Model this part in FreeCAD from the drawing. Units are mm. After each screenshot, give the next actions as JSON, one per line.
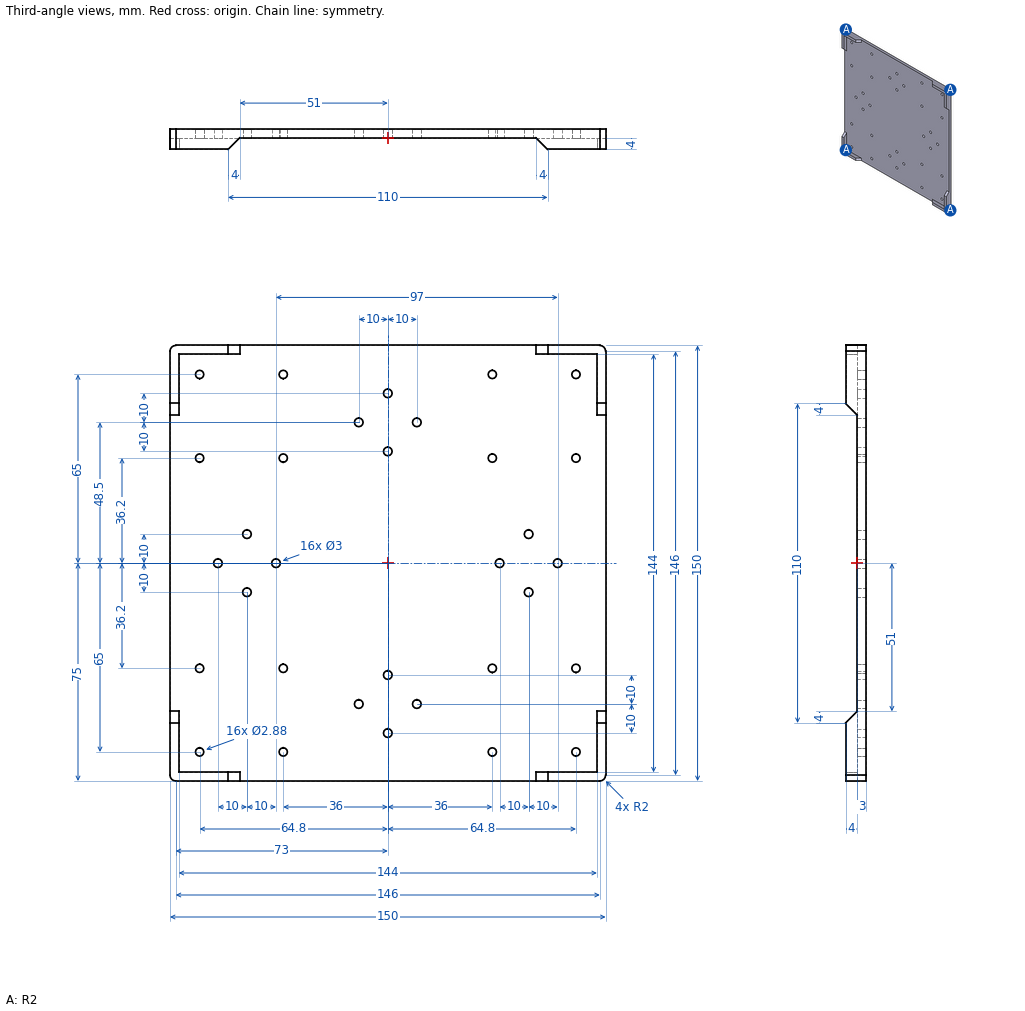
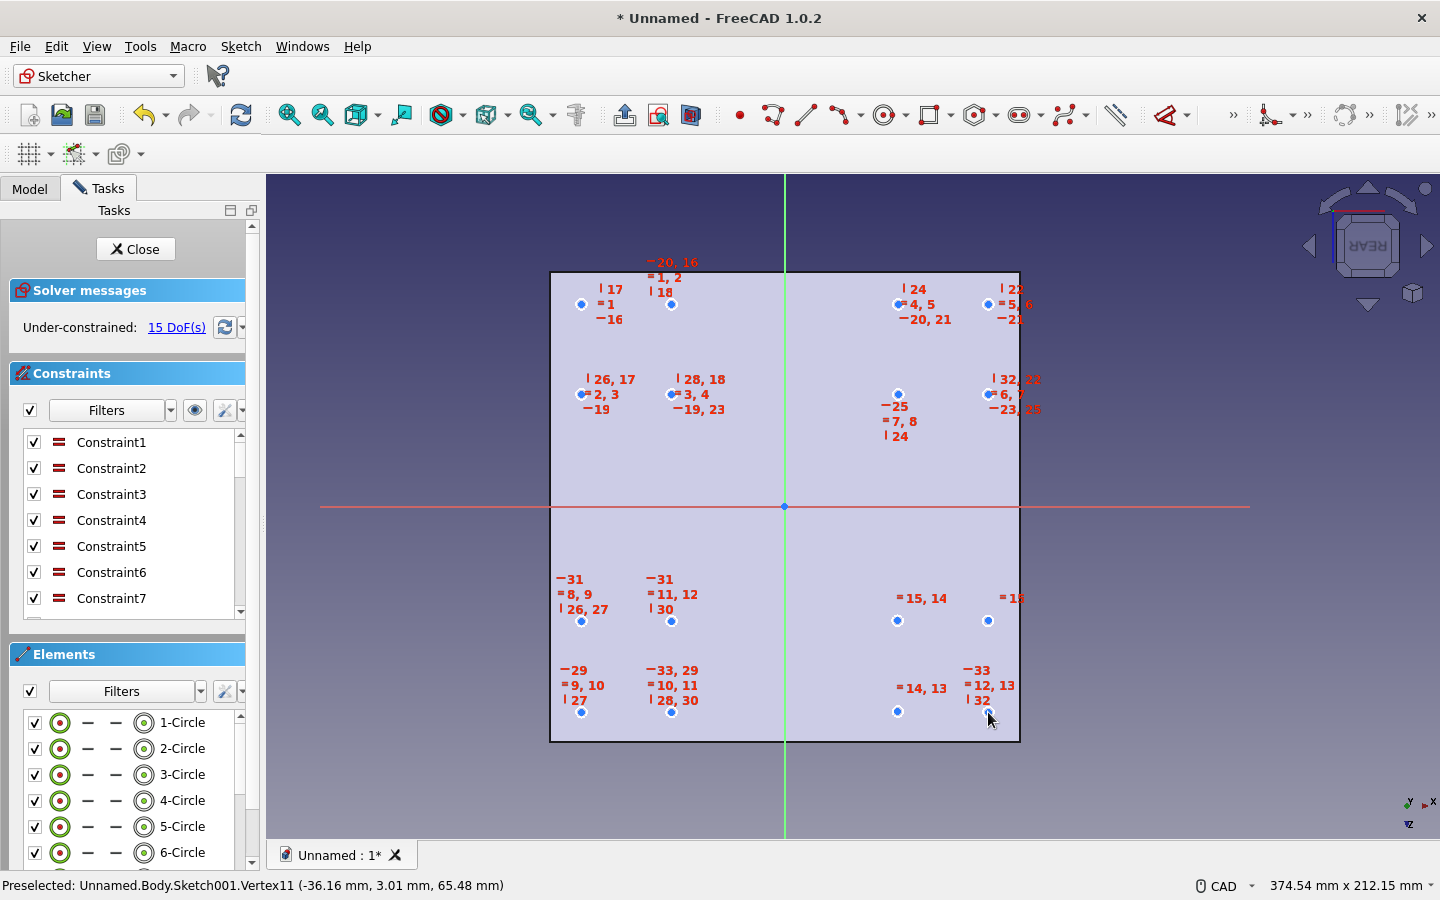
{"action": "left_click", "coordinate": [898, 394]}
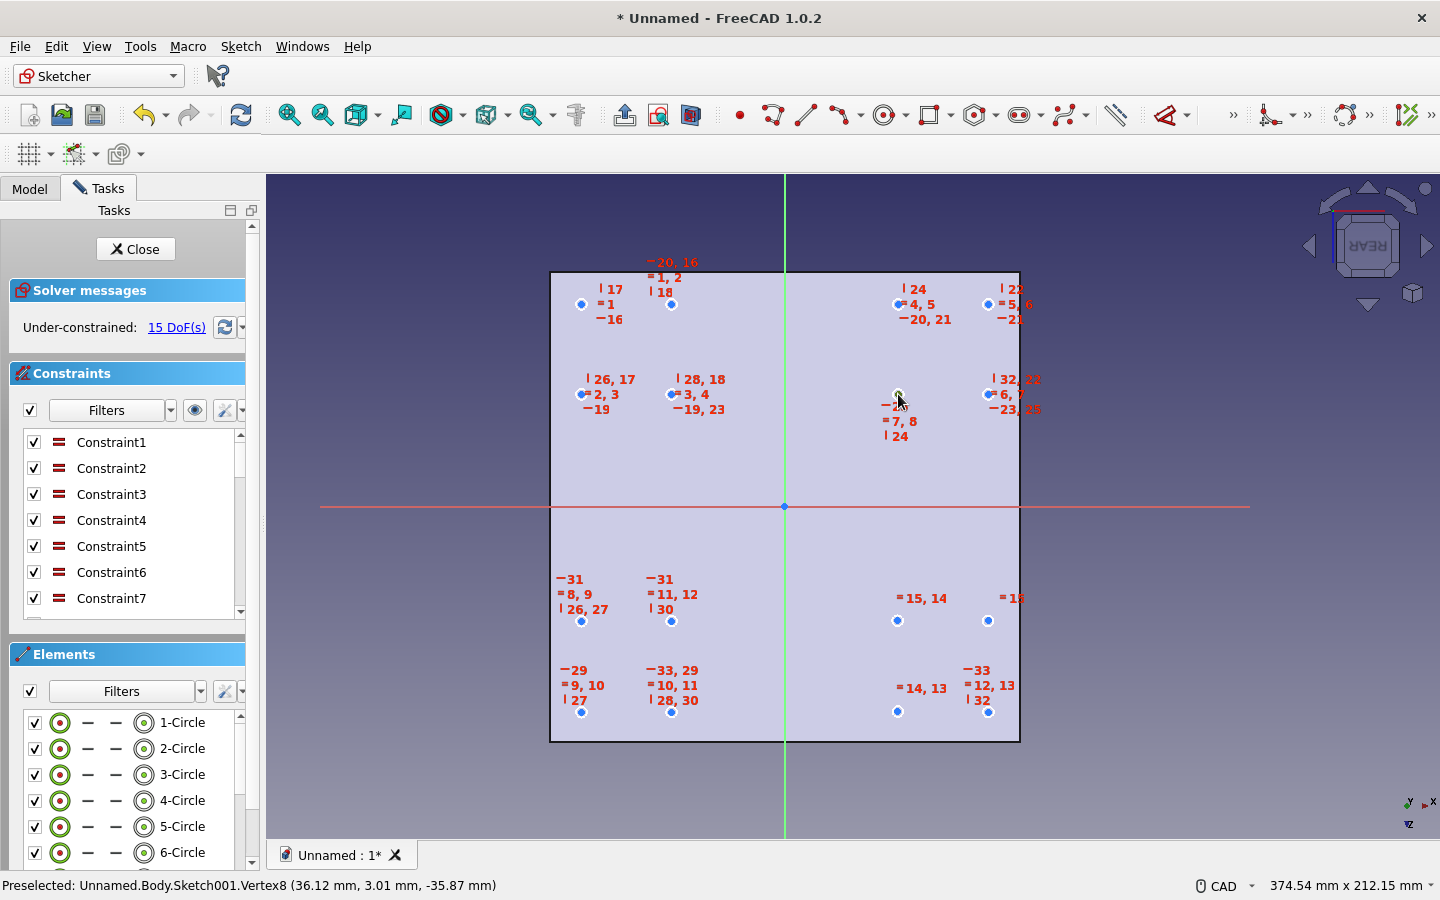
{"action": "left_click", "coordinate": [898, 712]}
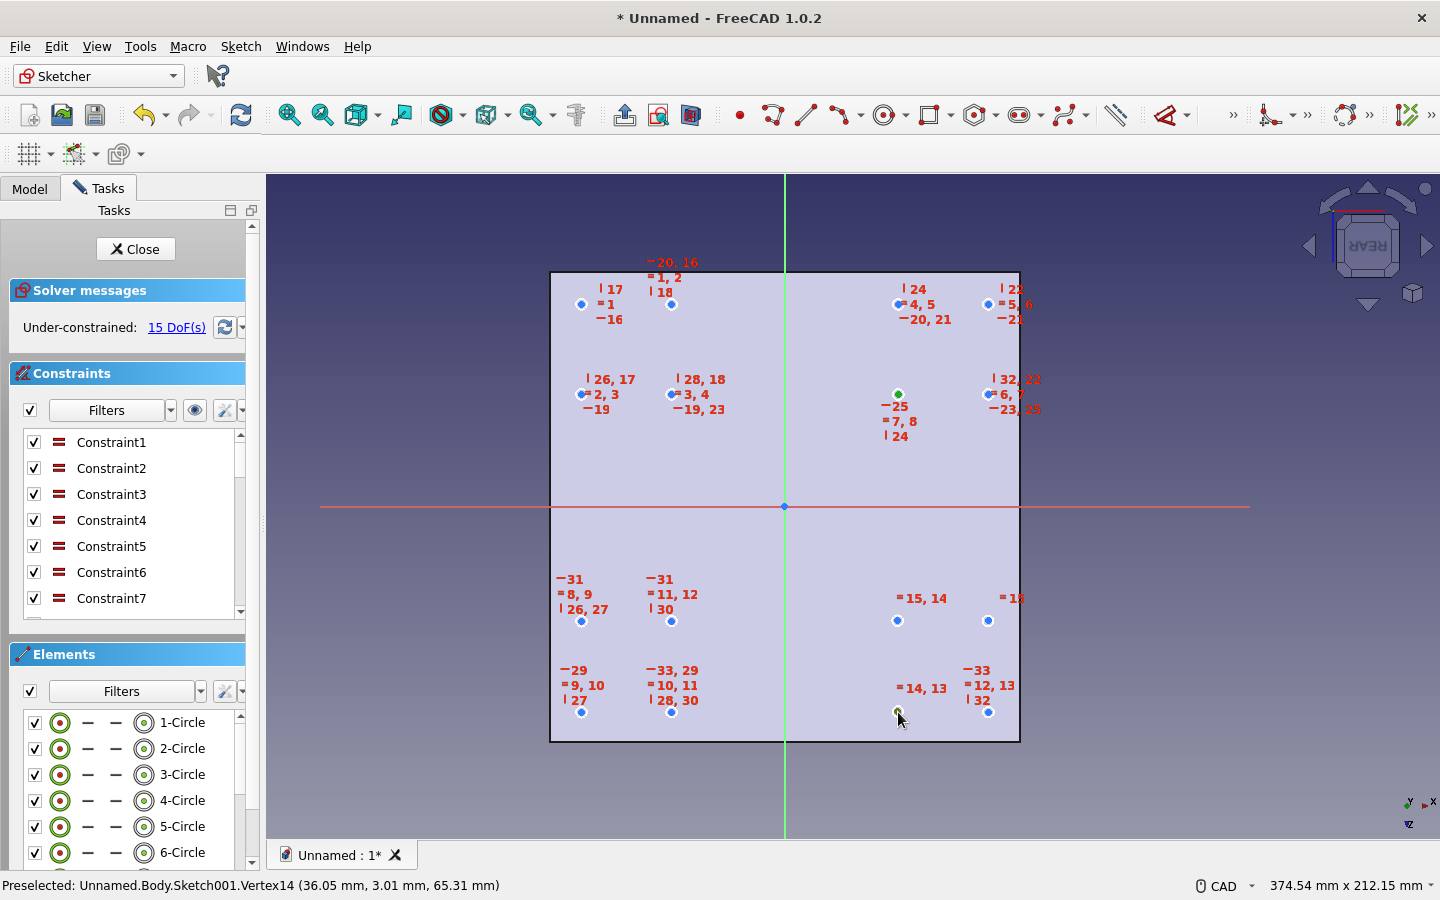
{"action": "key", "text": "v"}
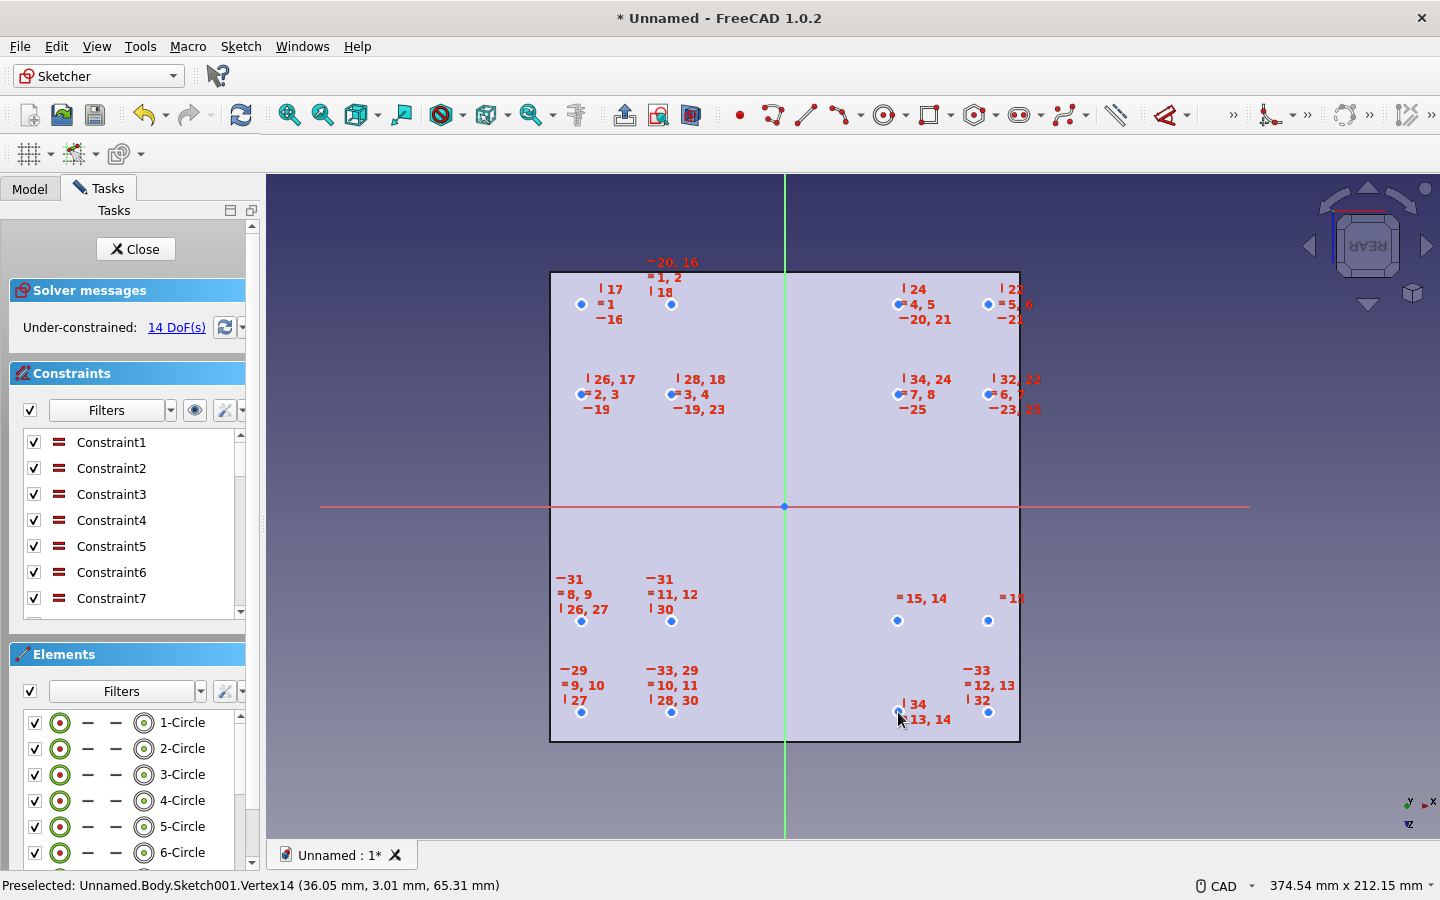
{"action": "left_click", "coordinate": [988, 712]}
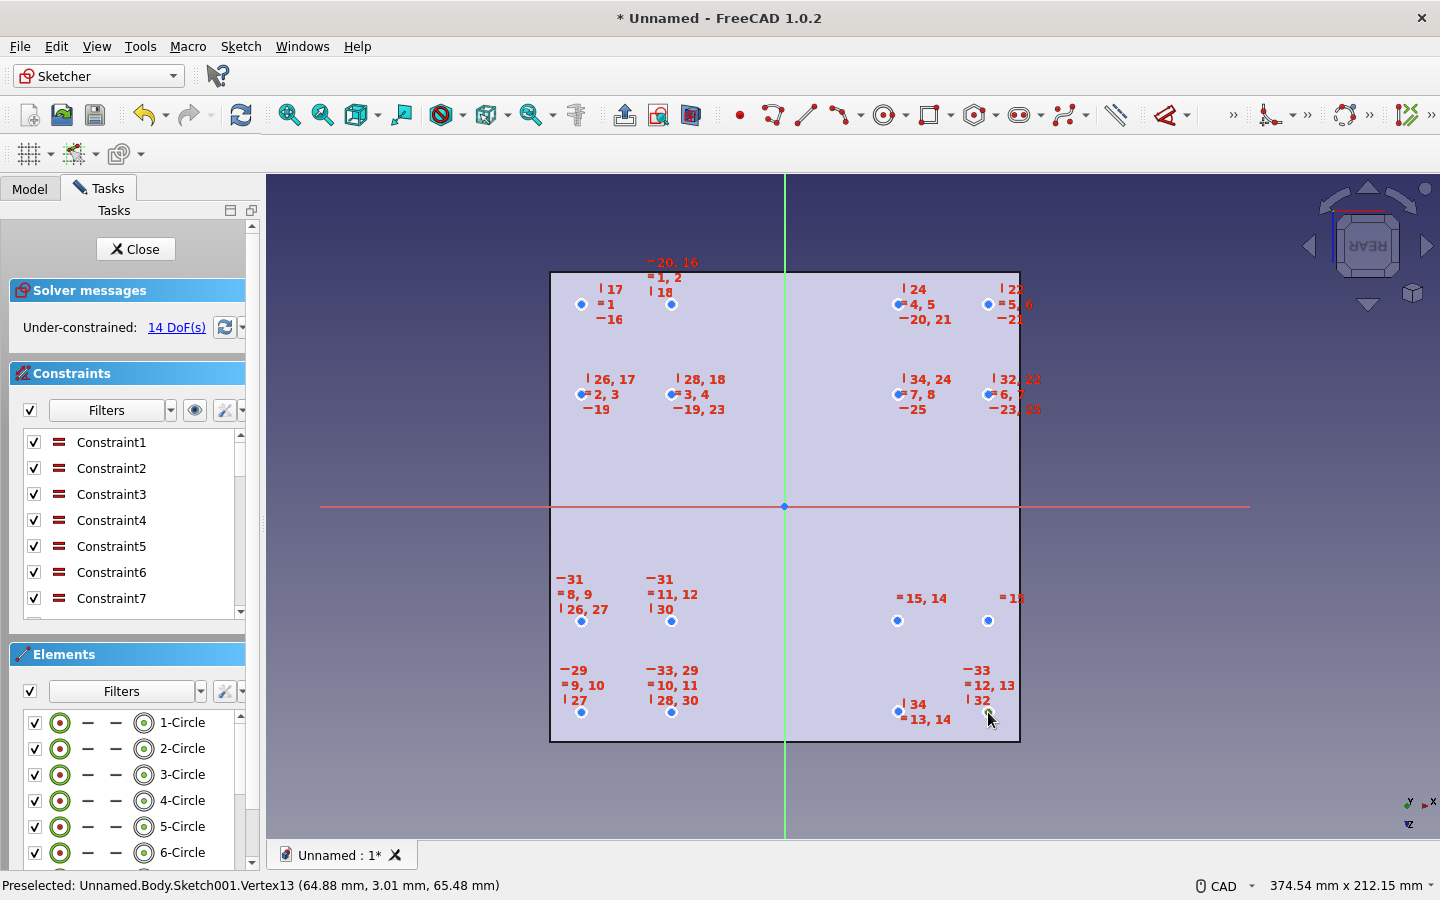
{"action": "left_click", "coordinate": [898, 712]}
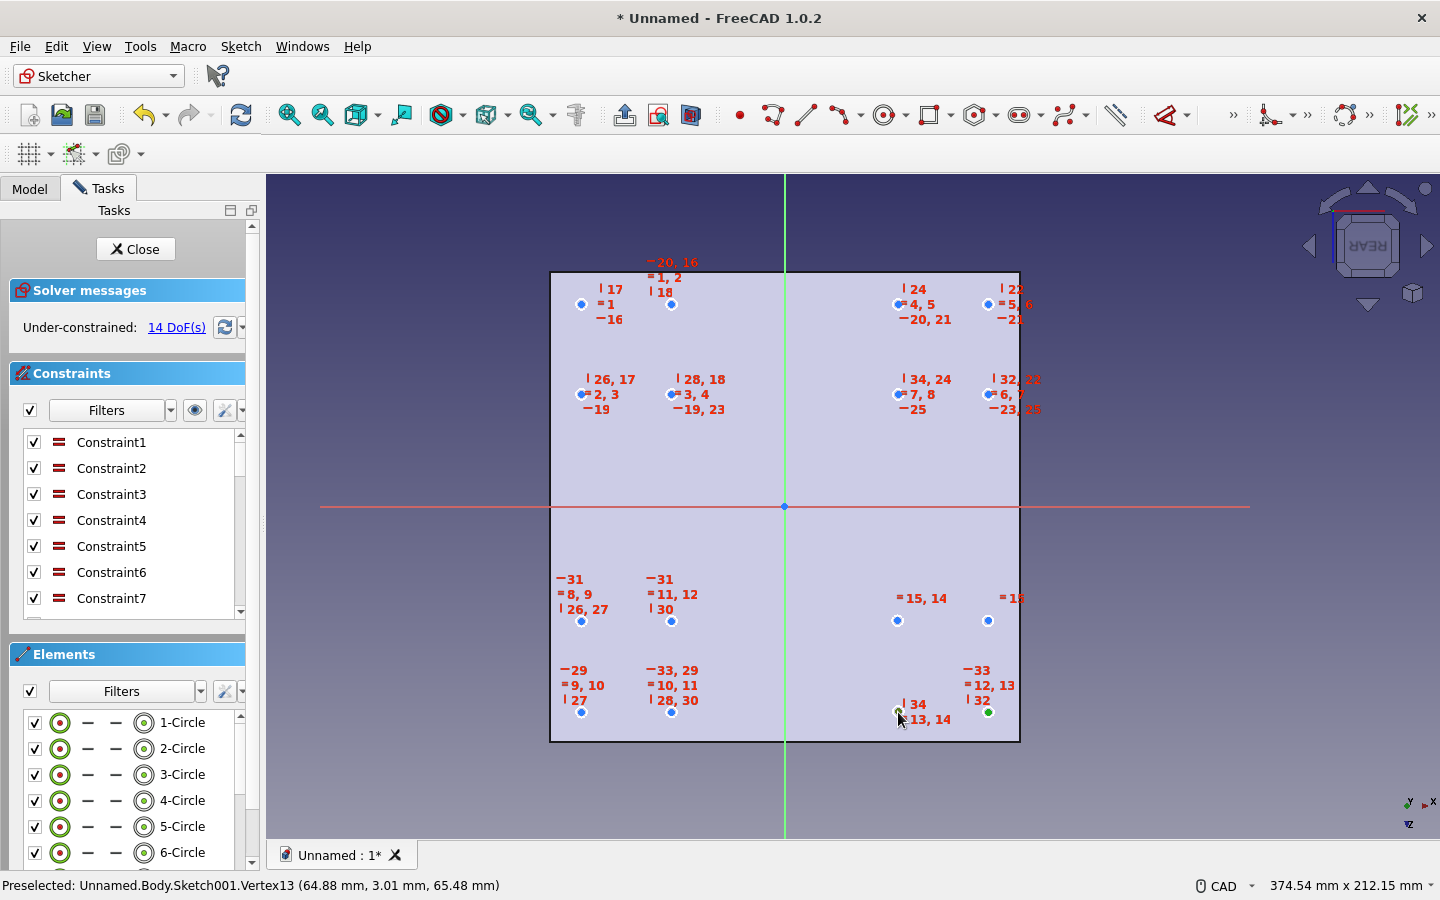
{"action": "key", "text": "h"}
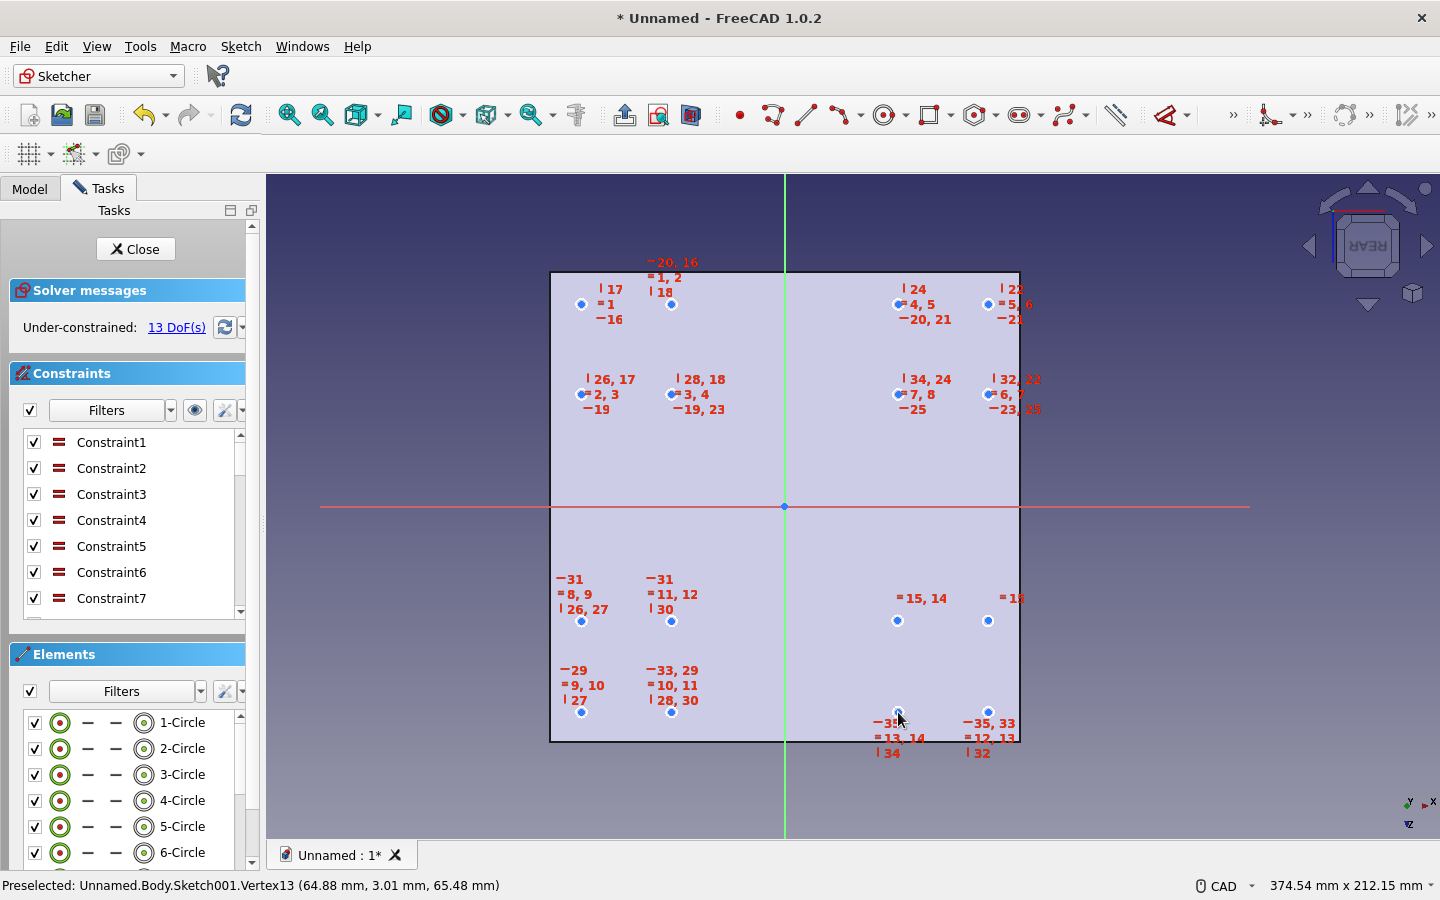
{"action": "left_click", "coordinate": [898, 712]}